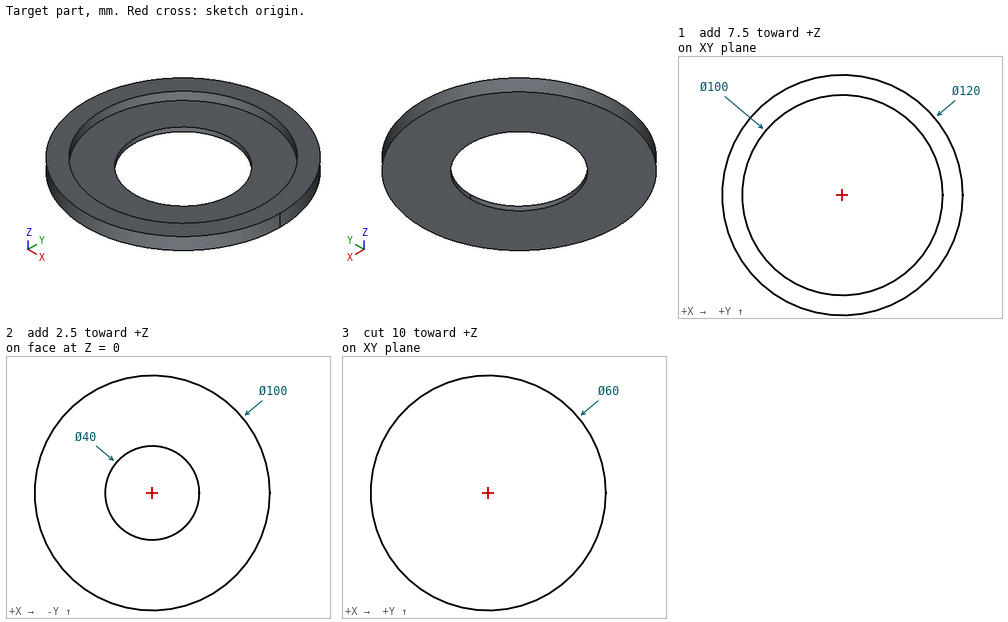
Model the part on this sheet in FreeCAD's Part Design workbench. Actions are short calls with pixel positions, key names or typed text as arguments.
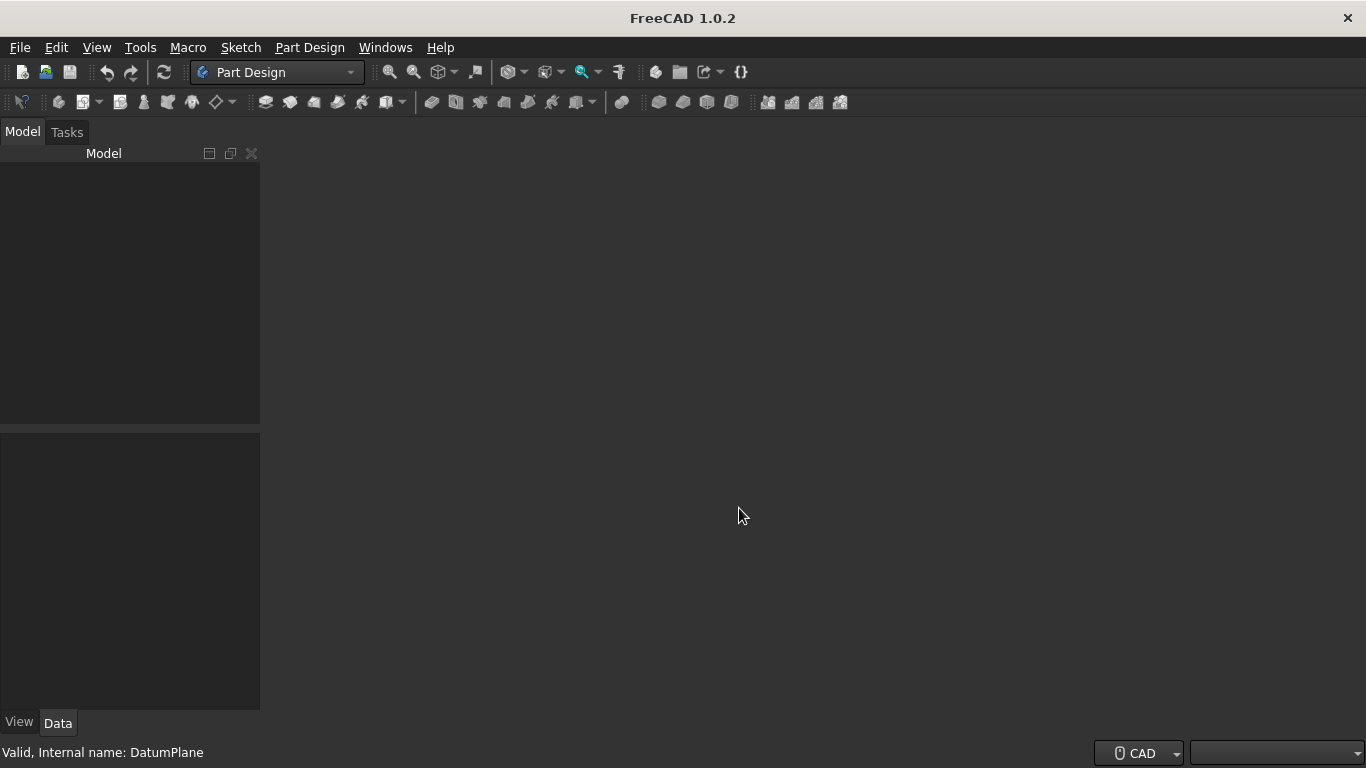
key(ctrl+n)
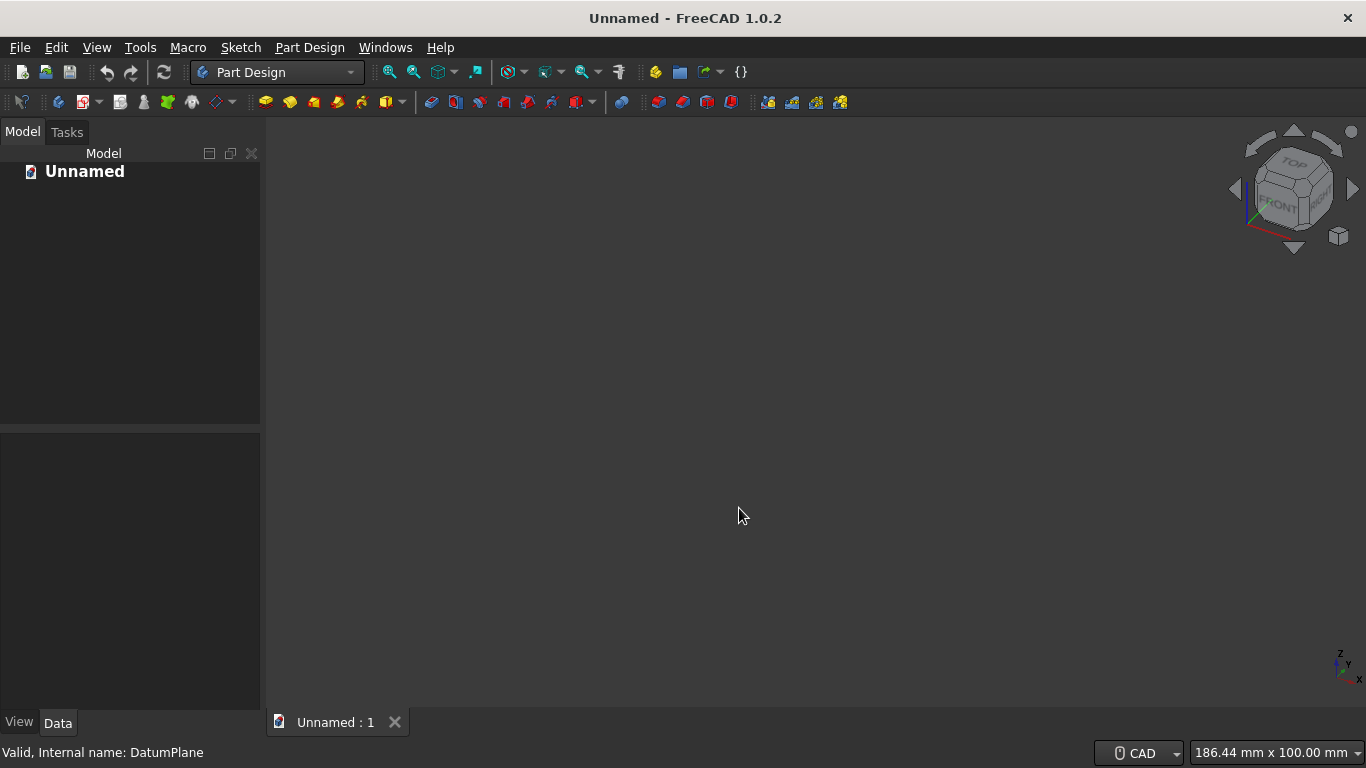
click(84, 102)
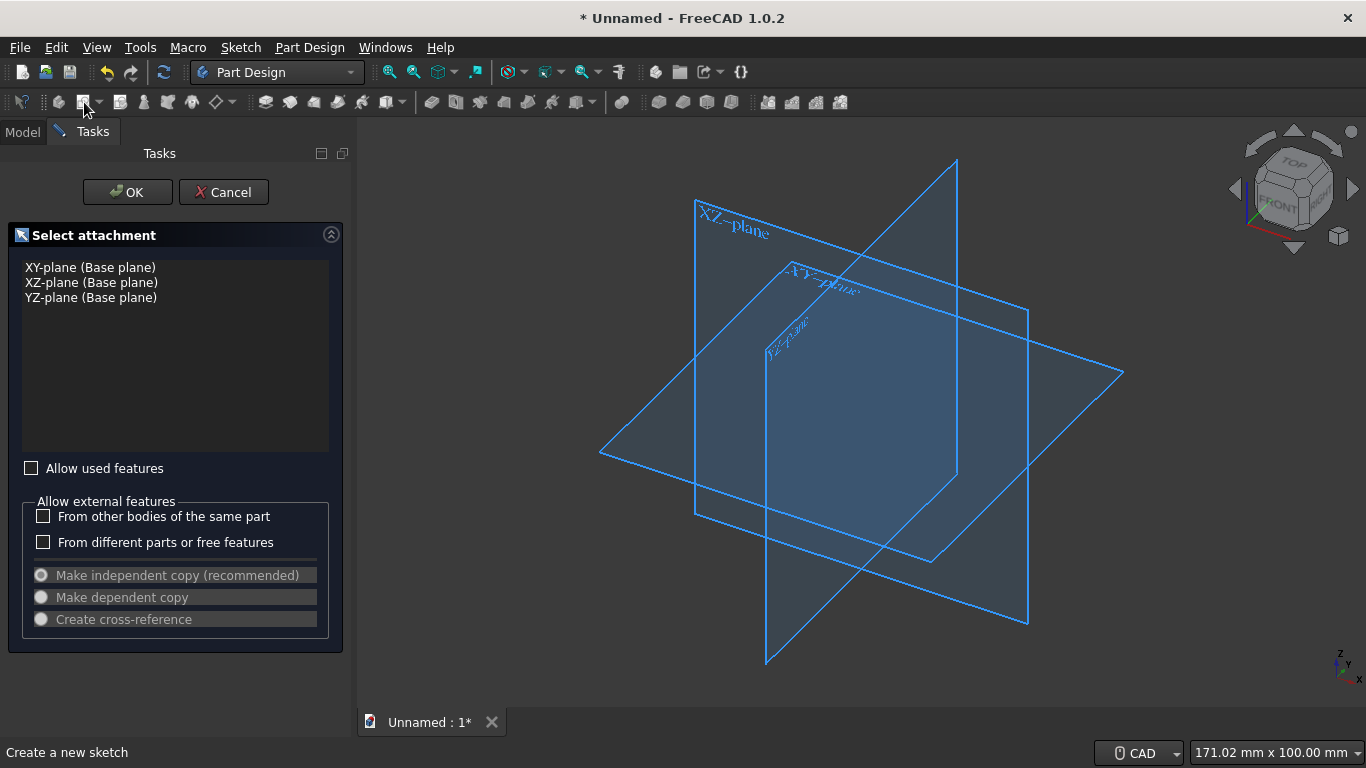
click(82, 268)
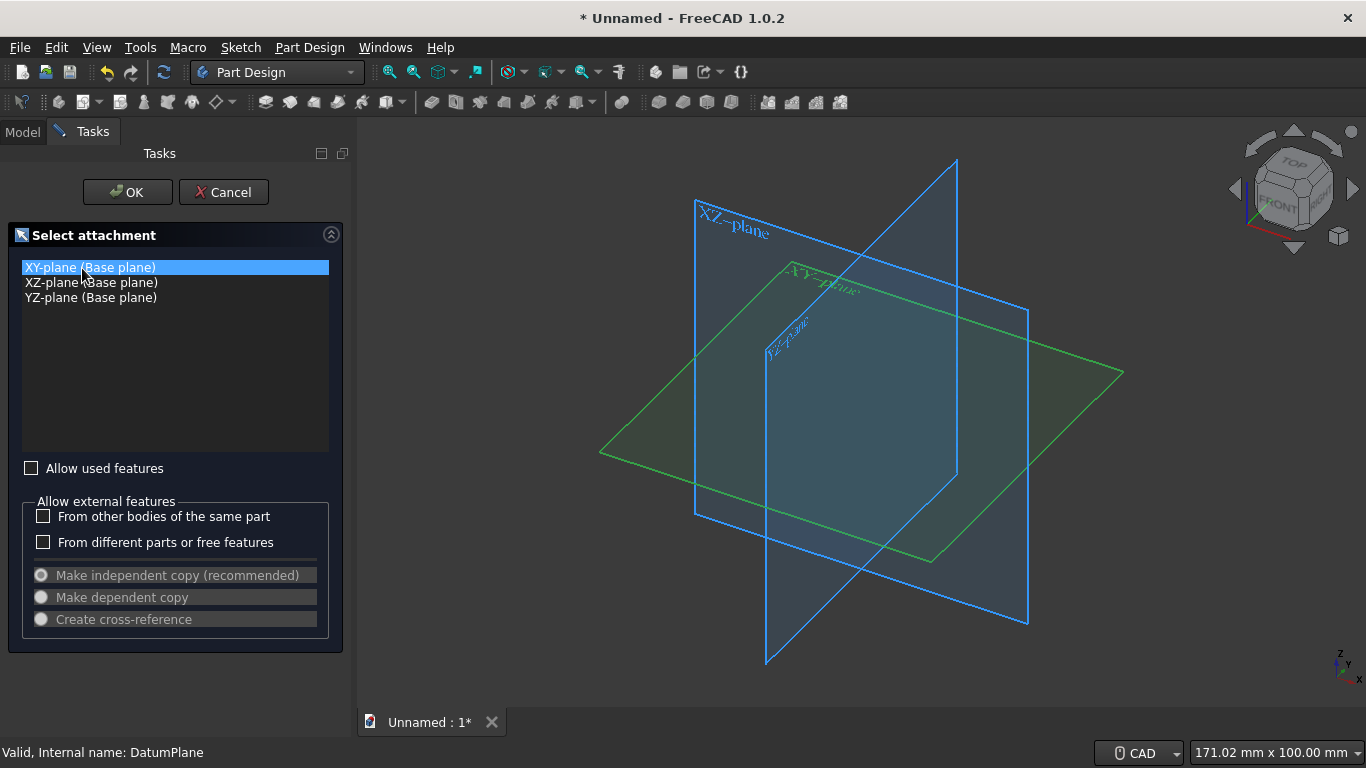
click(128, 192)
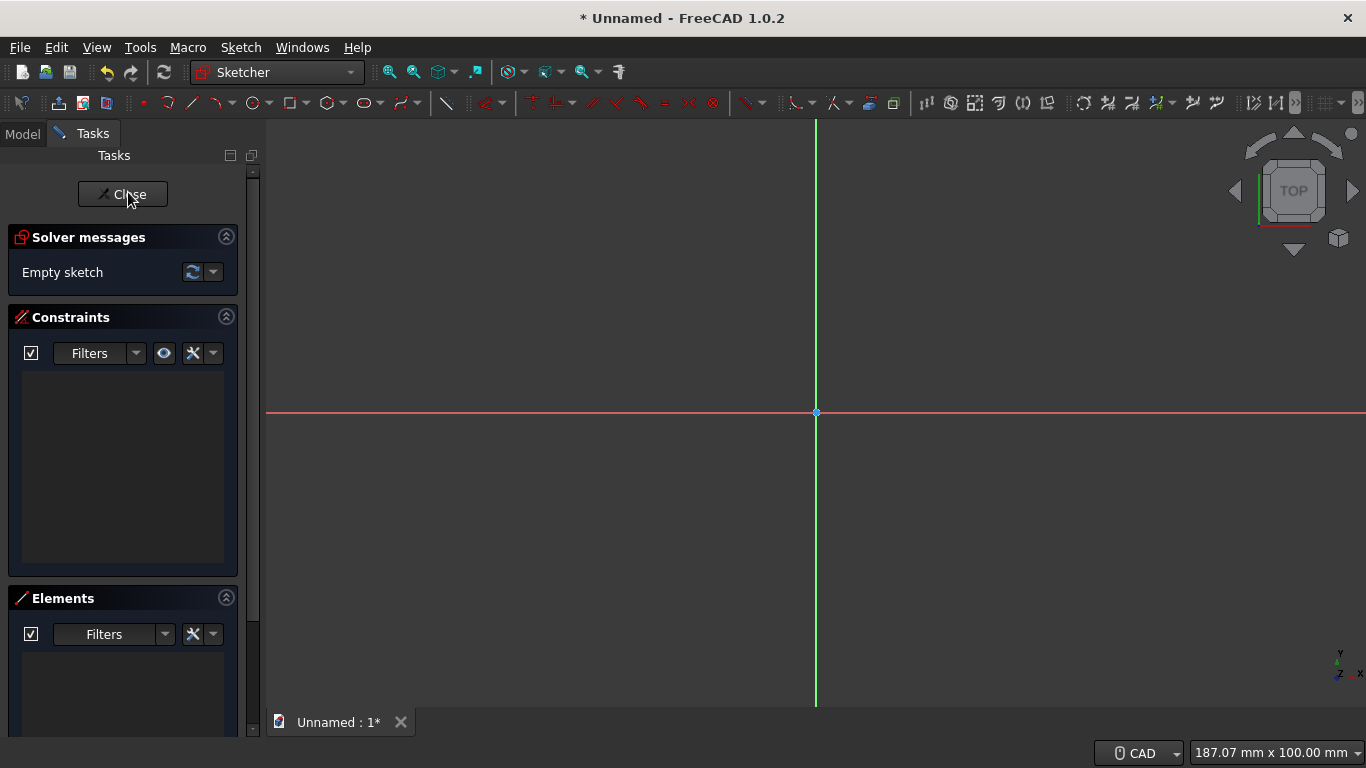
scroll(664, 413, down, 3)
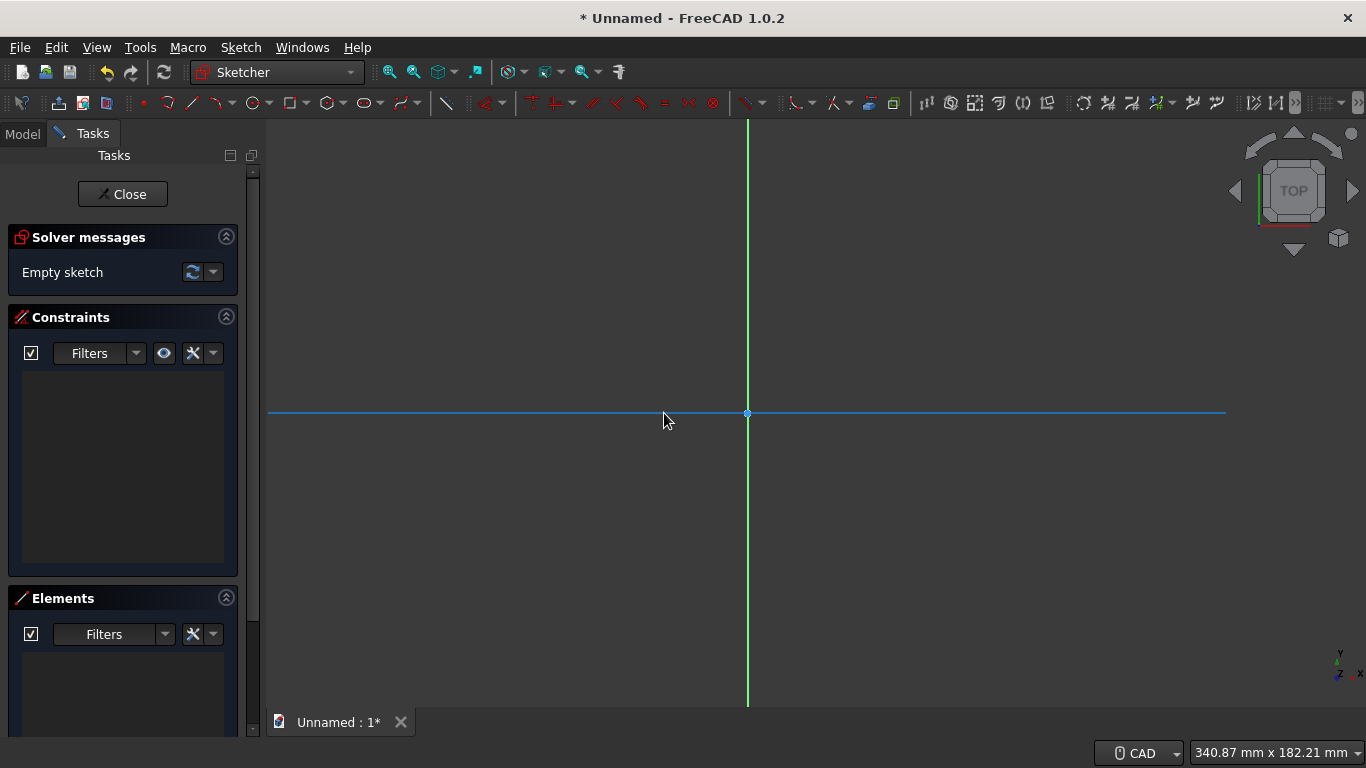
key(g)
key(c)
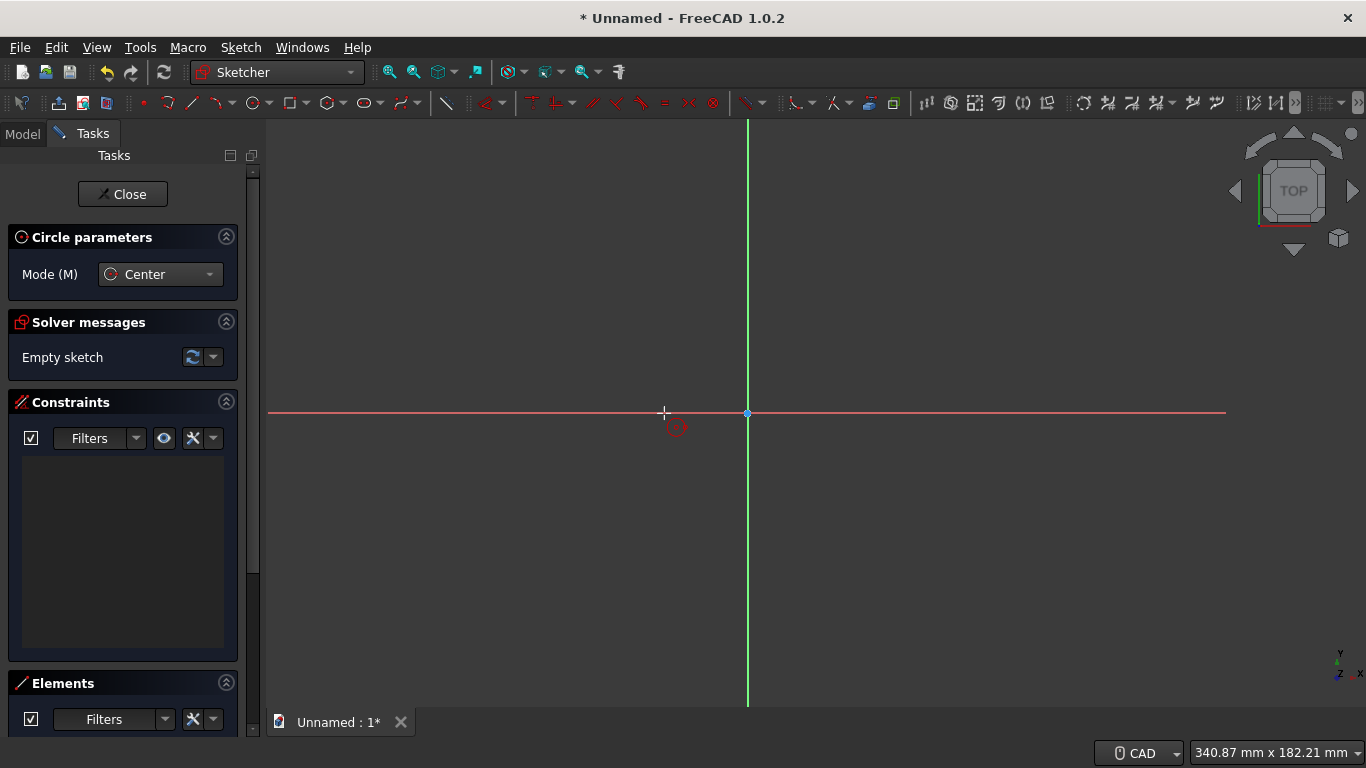
click(748, 413)
click(884, 276)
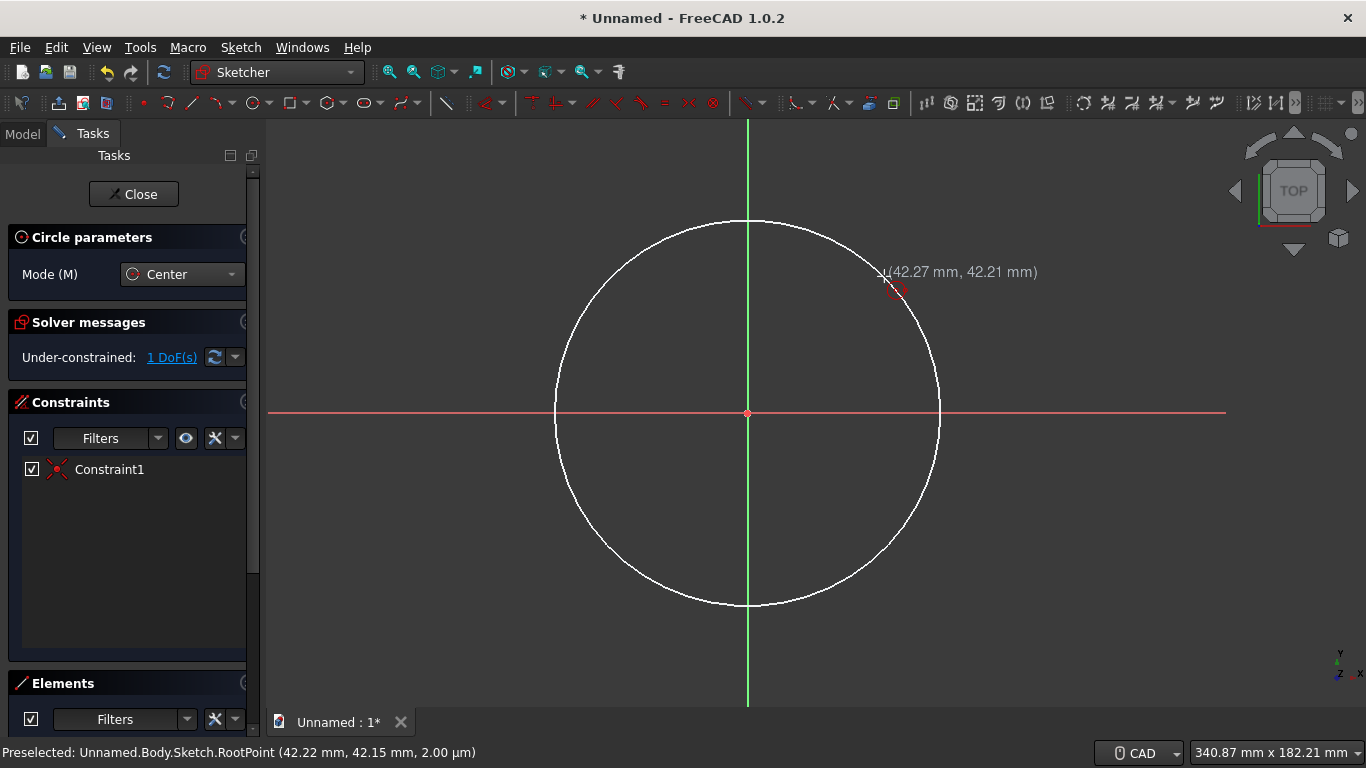
click(748, 413)
click(862, 299)
key(Escape)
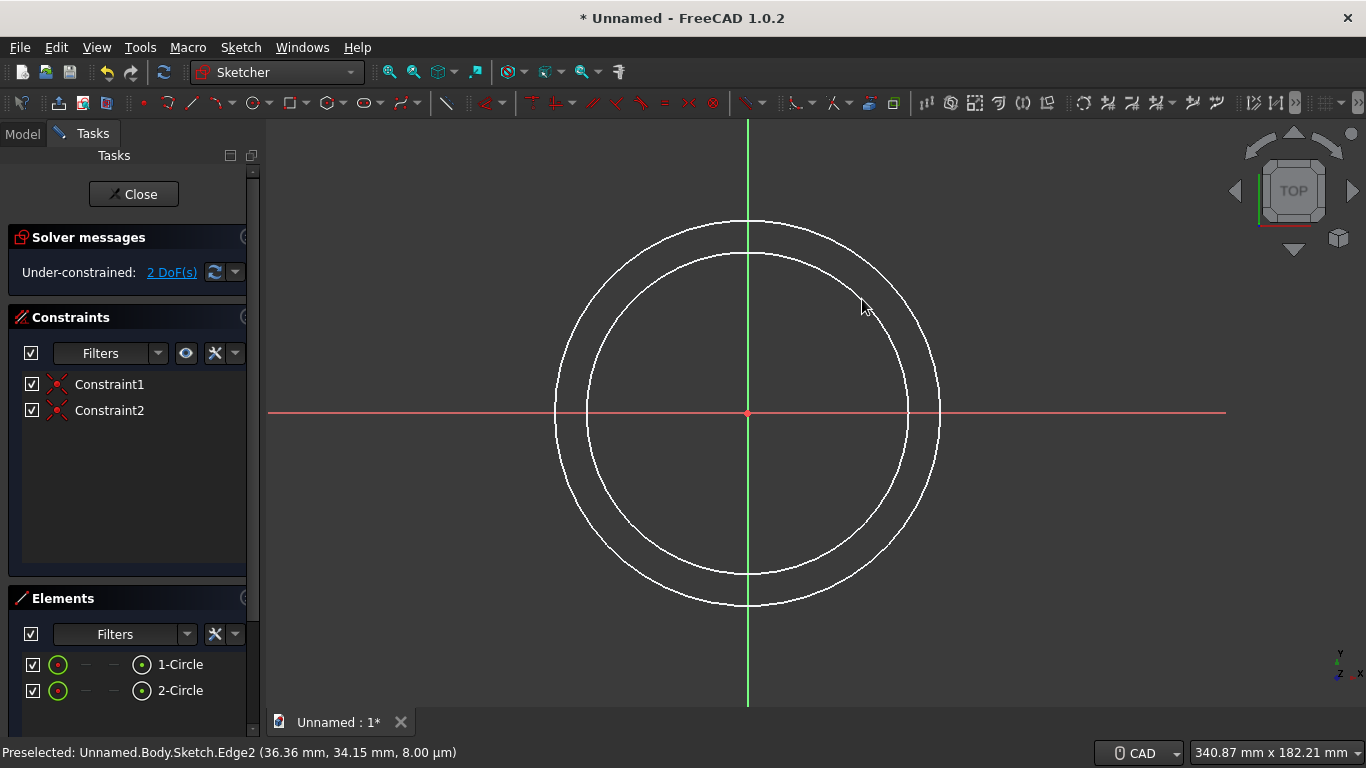
click(486, 104)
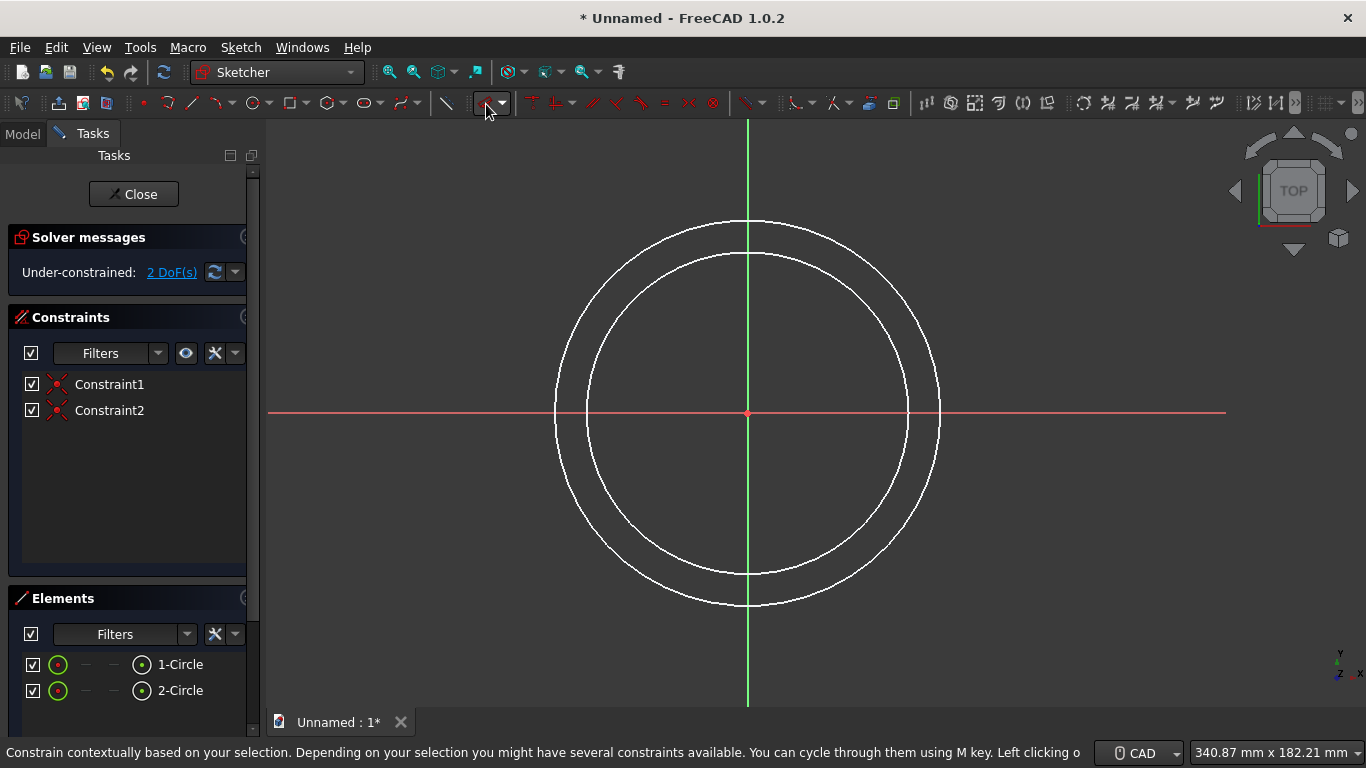
click(883, 276)
click(905, 253)